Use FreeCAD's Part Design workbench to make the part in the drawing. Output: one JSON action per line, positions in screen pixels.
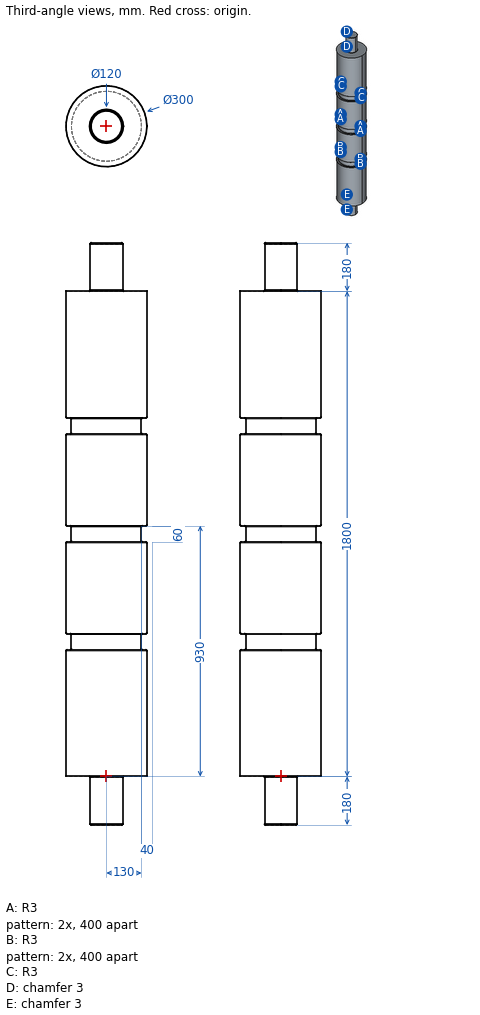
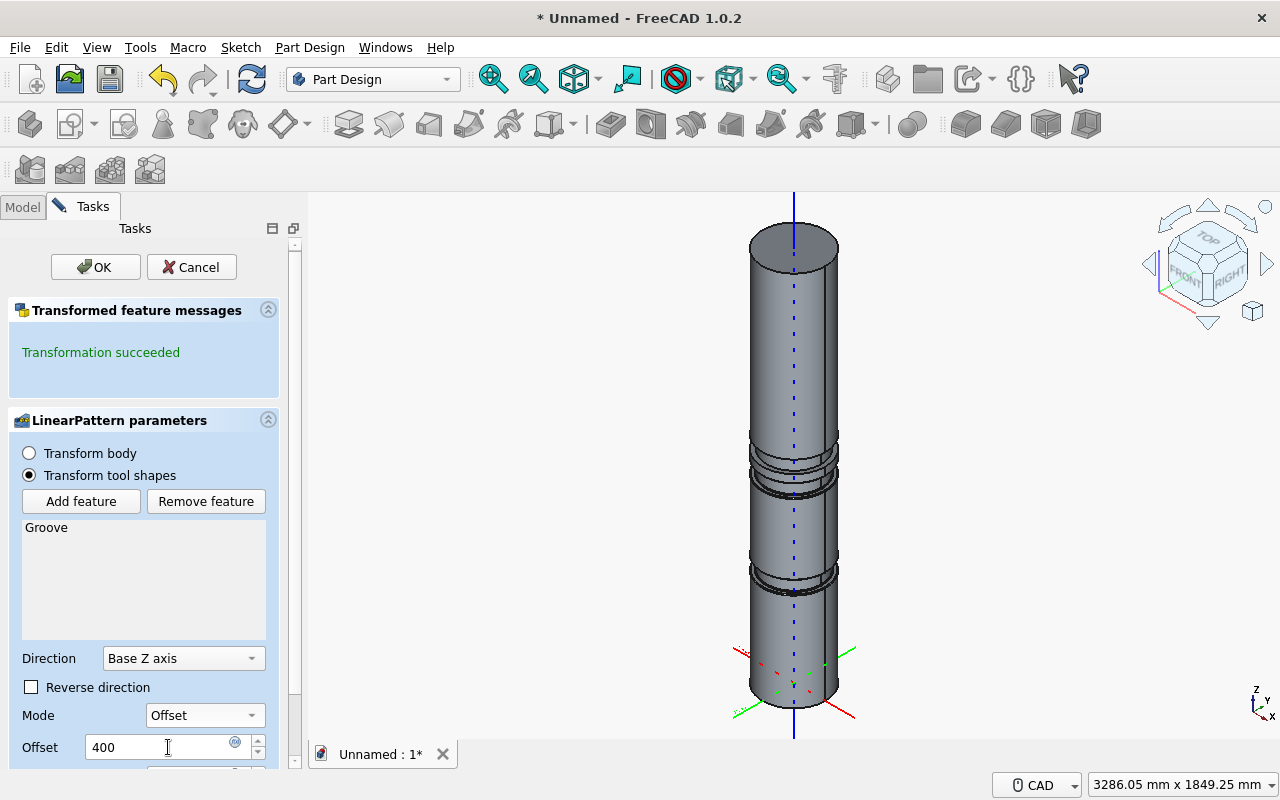
{"action": "scroll", "coordinate": [295, 503], "scroll_direction": "down", "scroll_amount": 2}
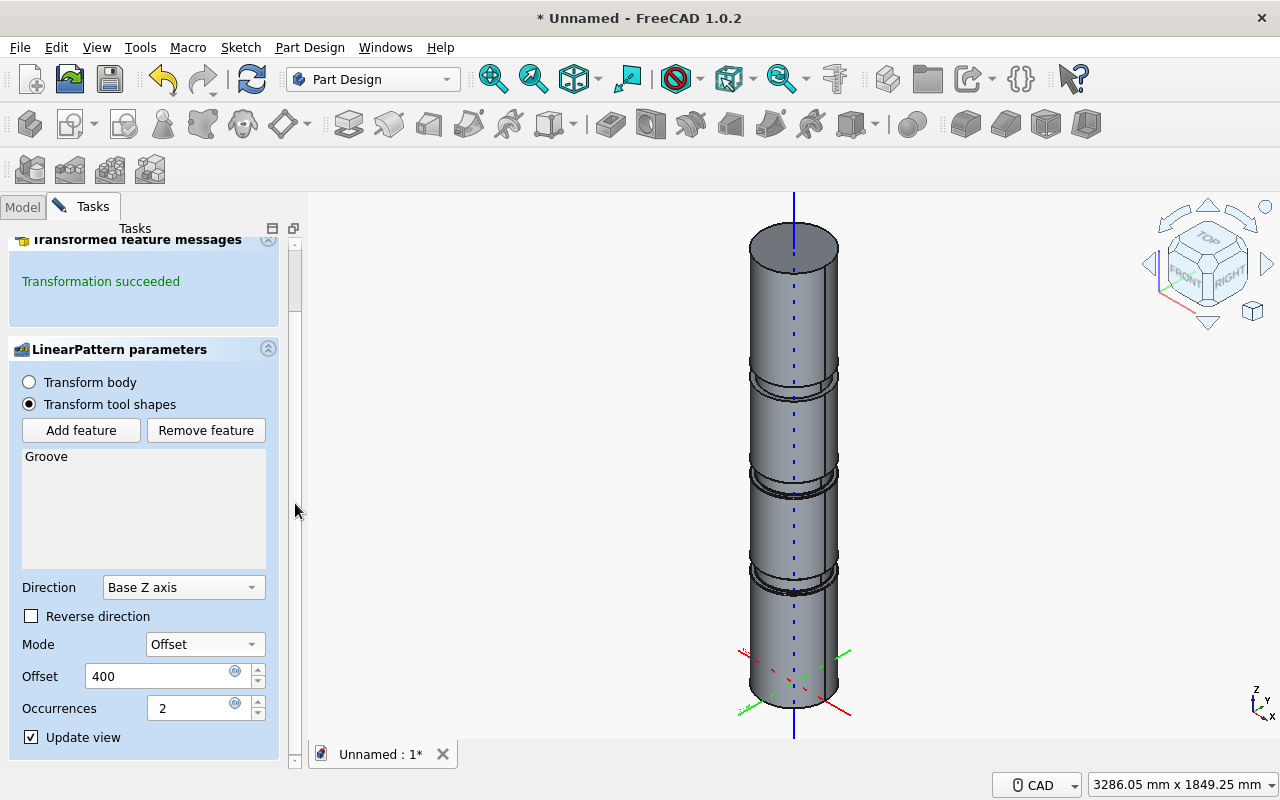
{"action": "triple_click", "coordinate": [198, 708]}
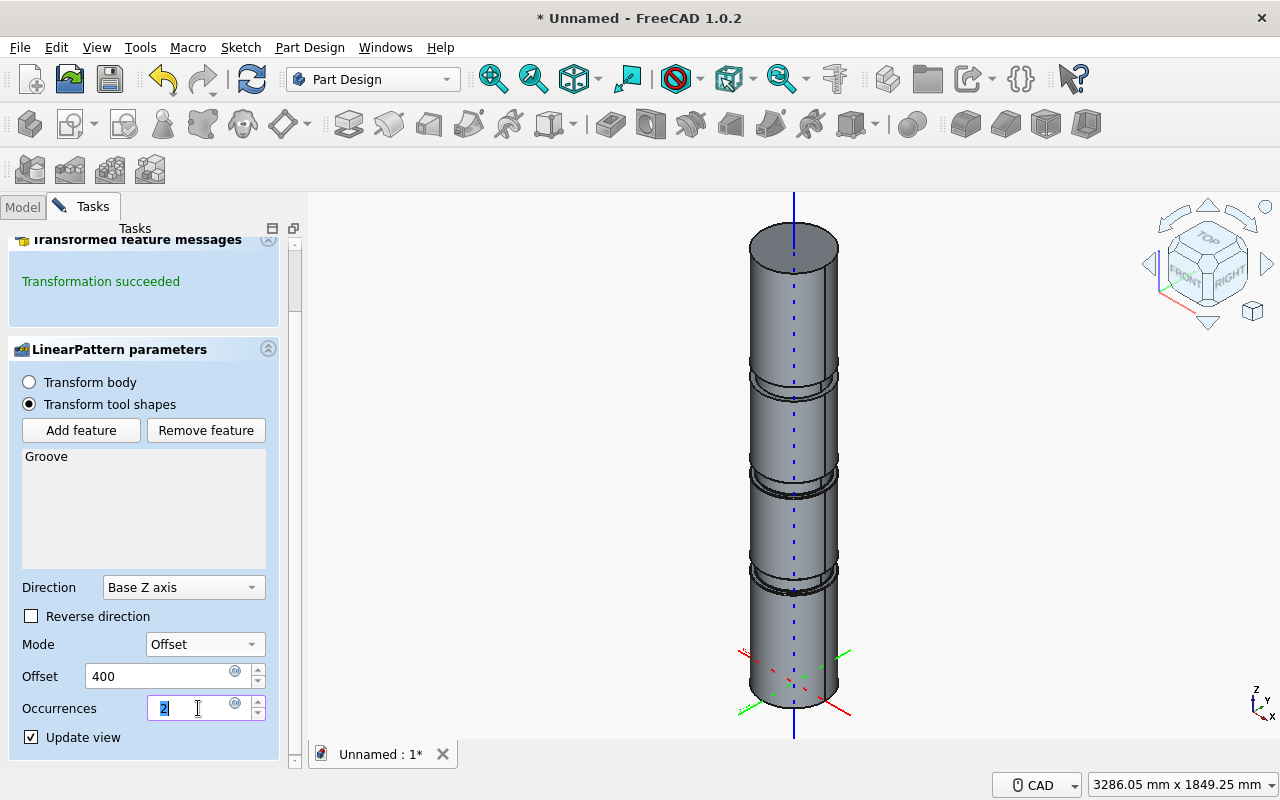
{"action": "type", "text": "2"}
{"action": "key", "text": "Tab"}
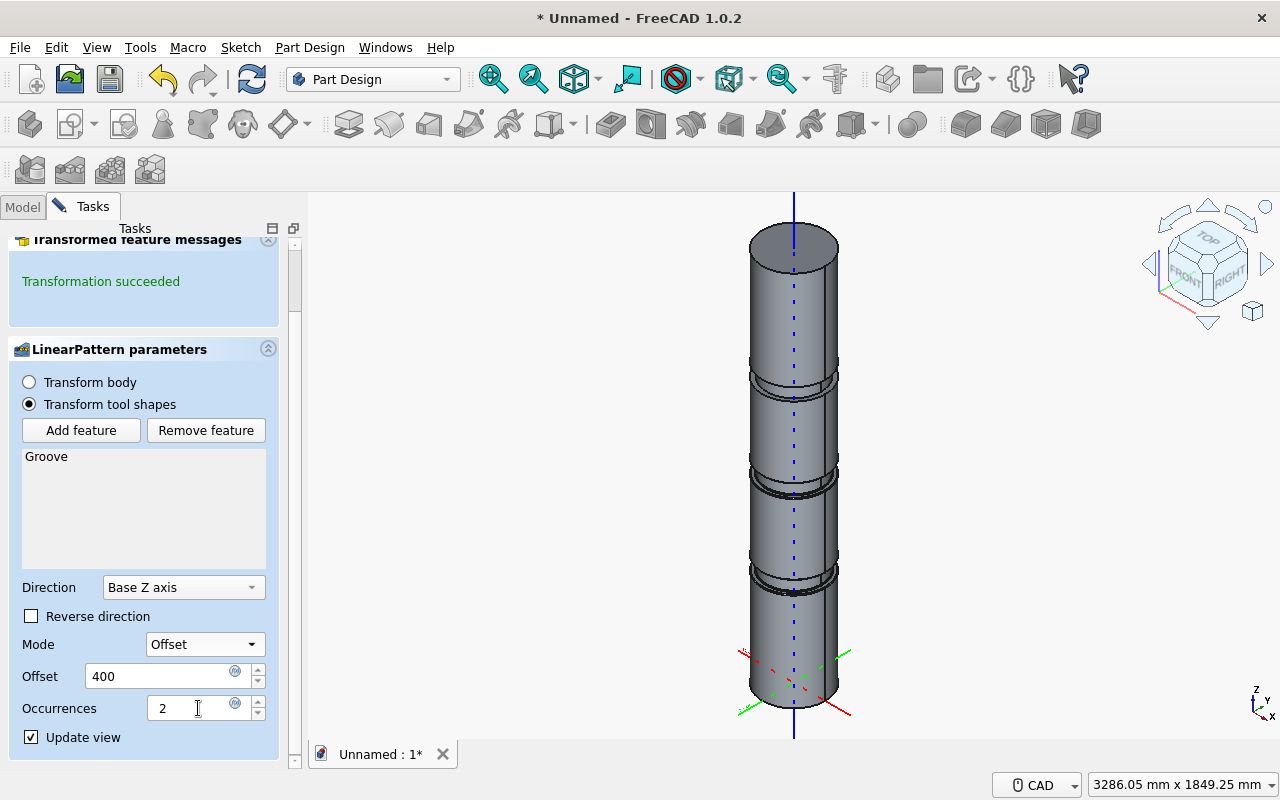
{"action": "scroll", "coordinate": [295, 503], "scroll_direction": "up", "scroll_amount": 2}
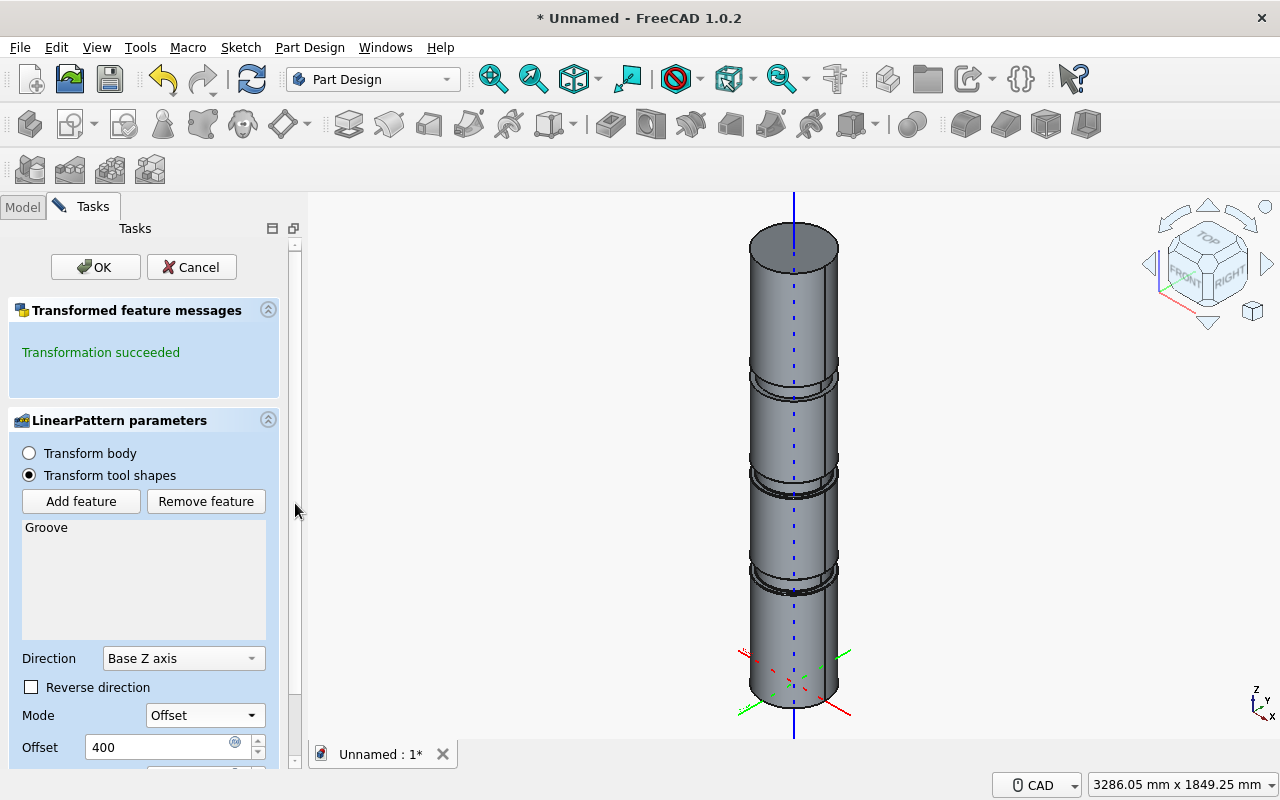
{"action": "left_click", "coordinate": [96, 267]}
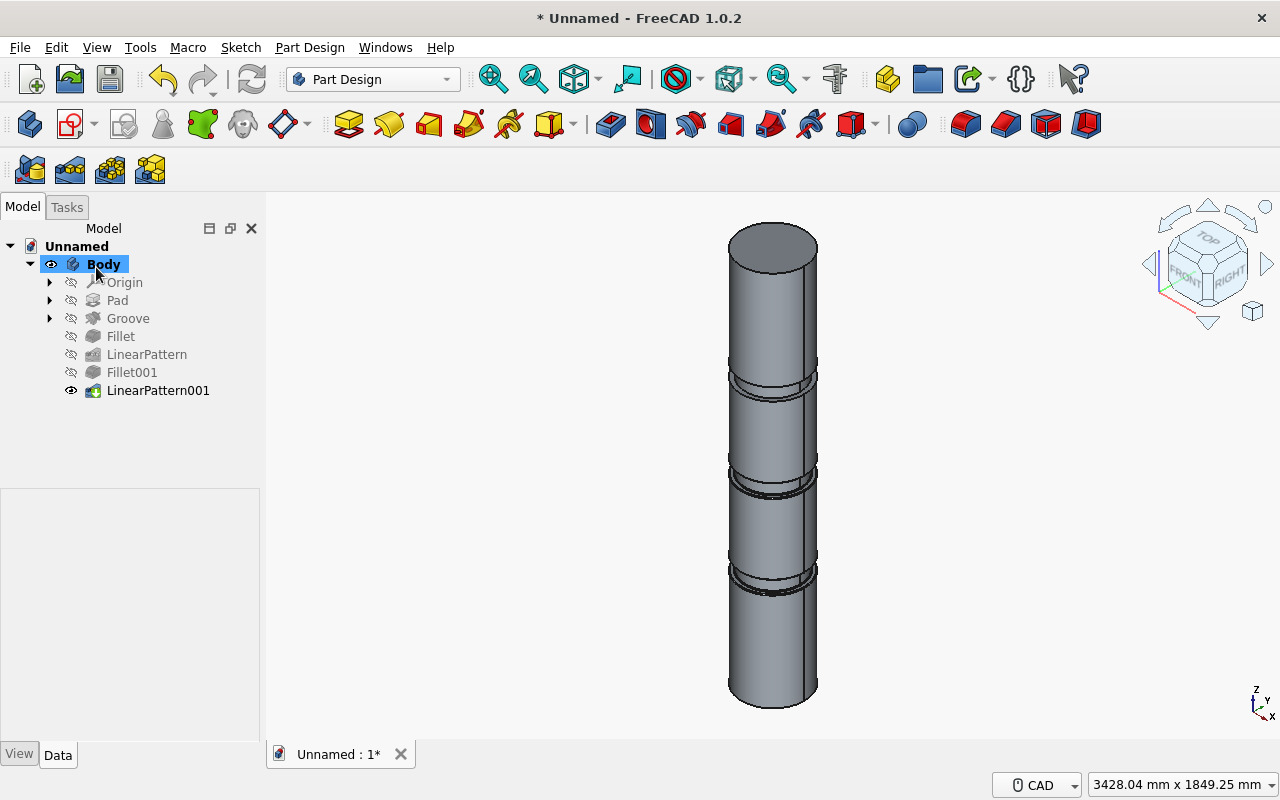
{"action": "left_click", "coordinate": [733, 372]}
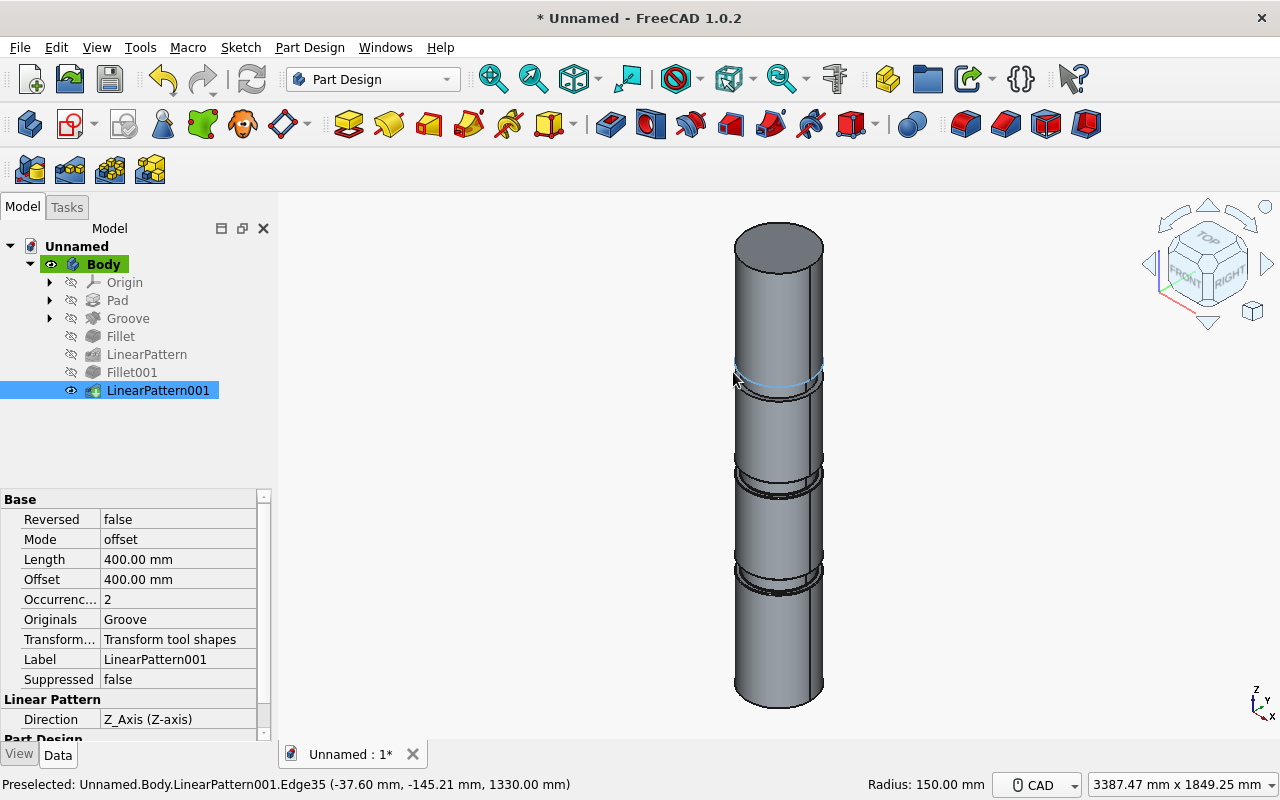
{"action": "left_click", "coordinate": [739, 387], "text": "ctrl"}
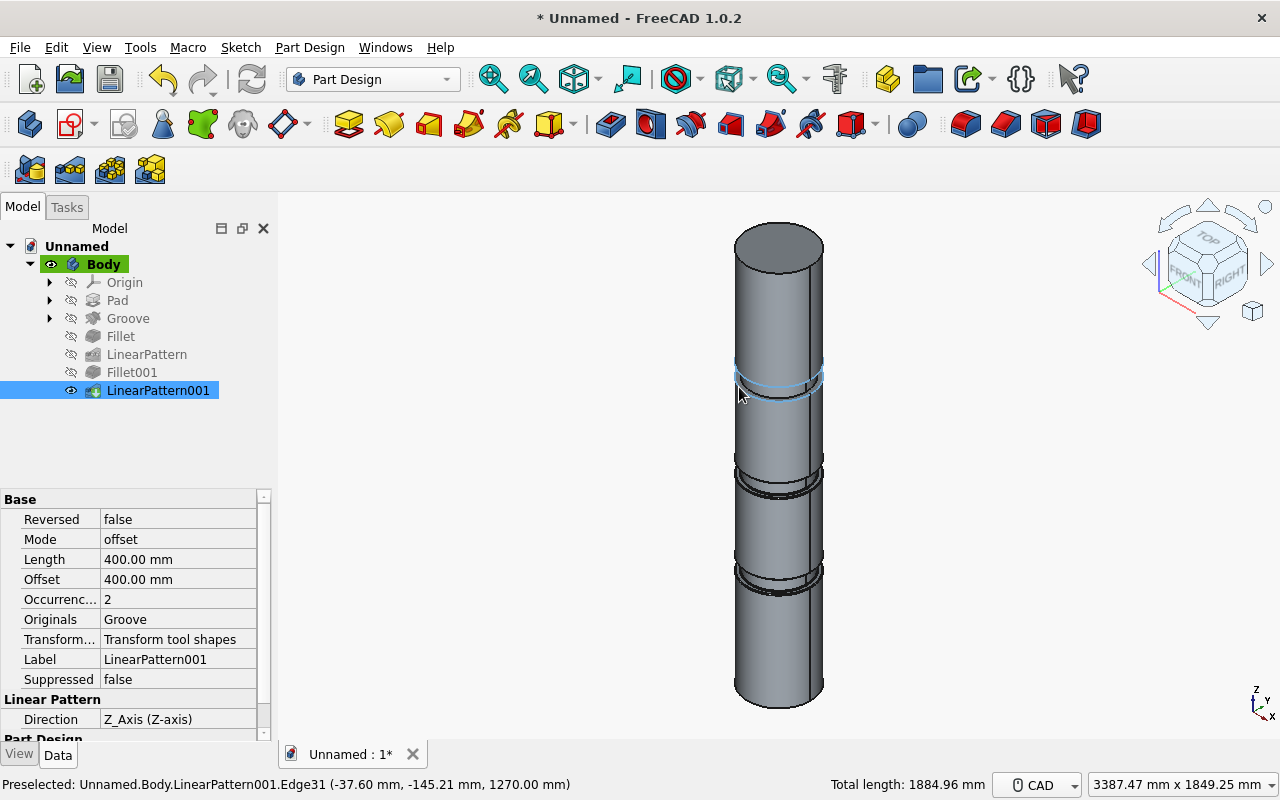
{"action": "key", "text": "2"}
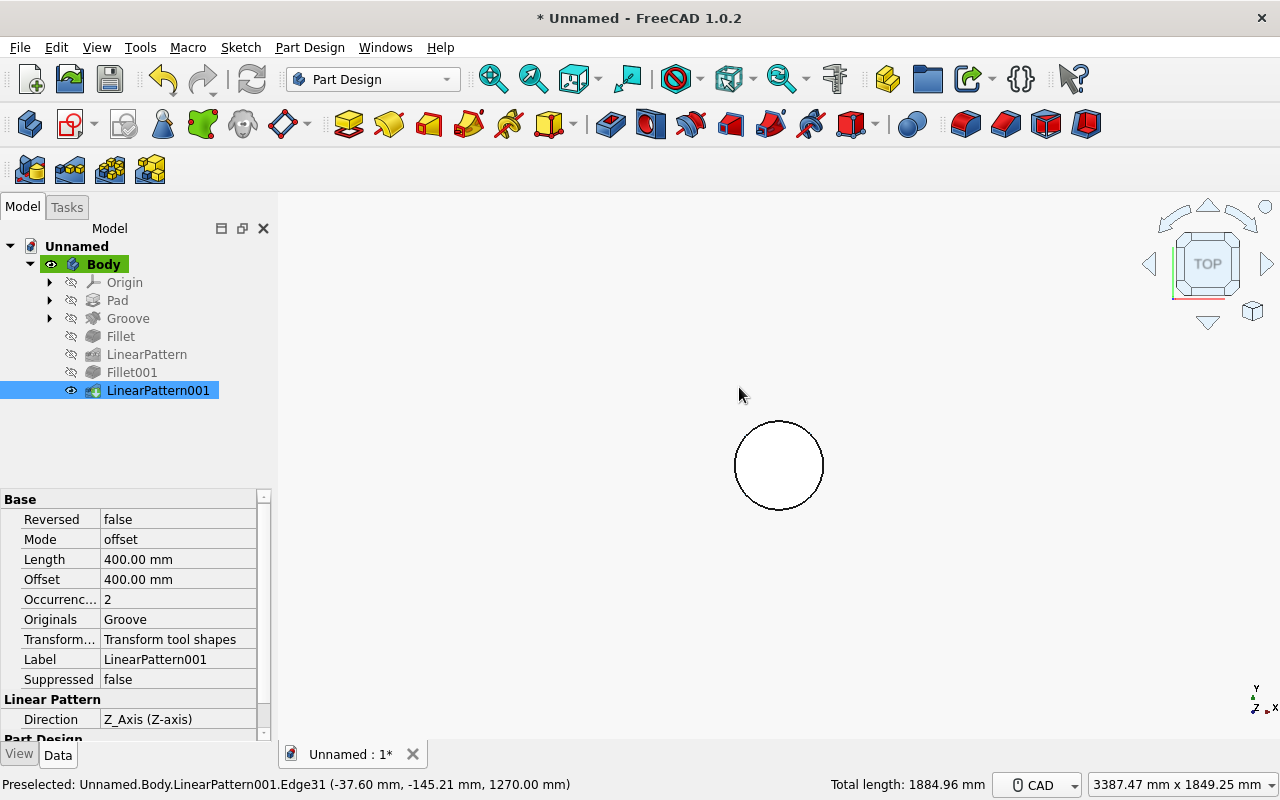
{"action": "left_click", "coordinate": [494, 80]}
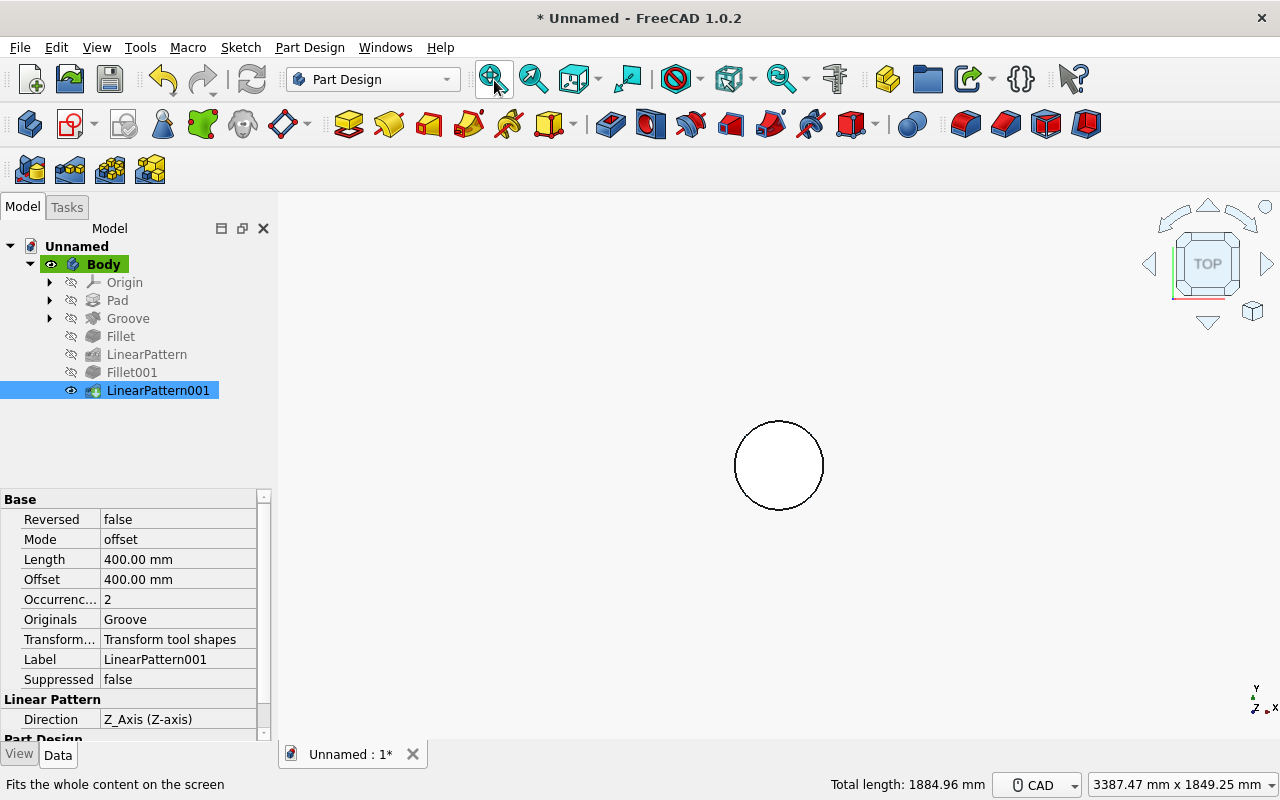
{"action": "key", "text": "0"}